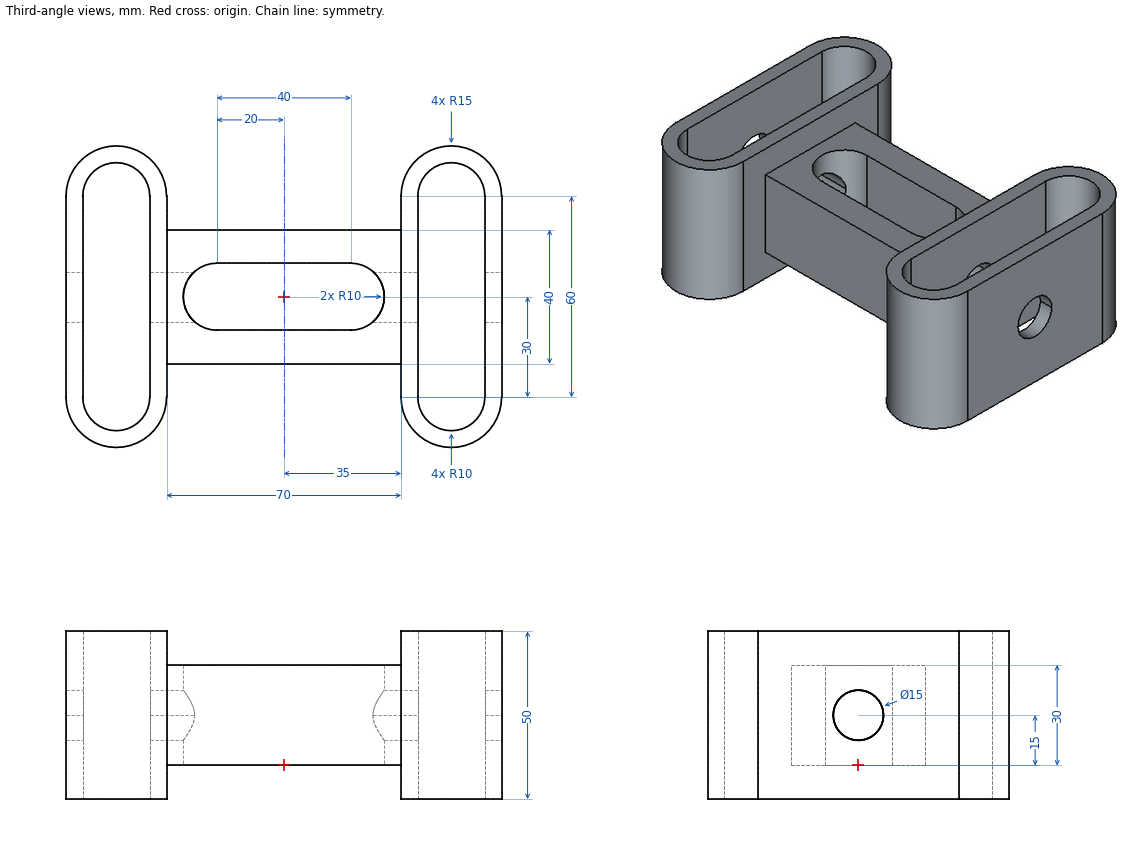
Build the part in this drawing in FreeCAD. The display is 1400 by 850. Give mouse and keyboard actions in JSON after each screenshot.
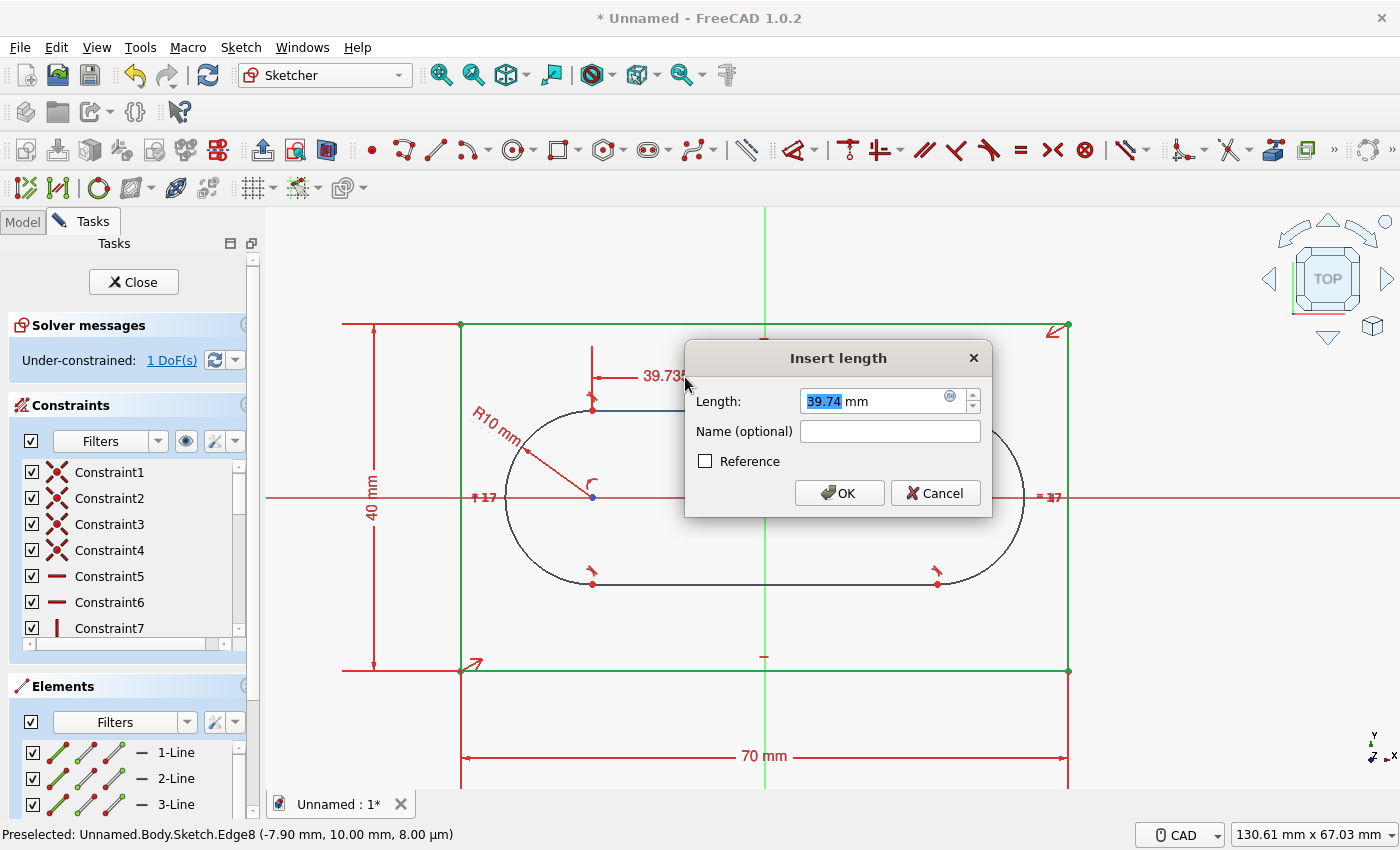
{"action": "type", "text": "40"}
{"action": "key", "text": "Return"}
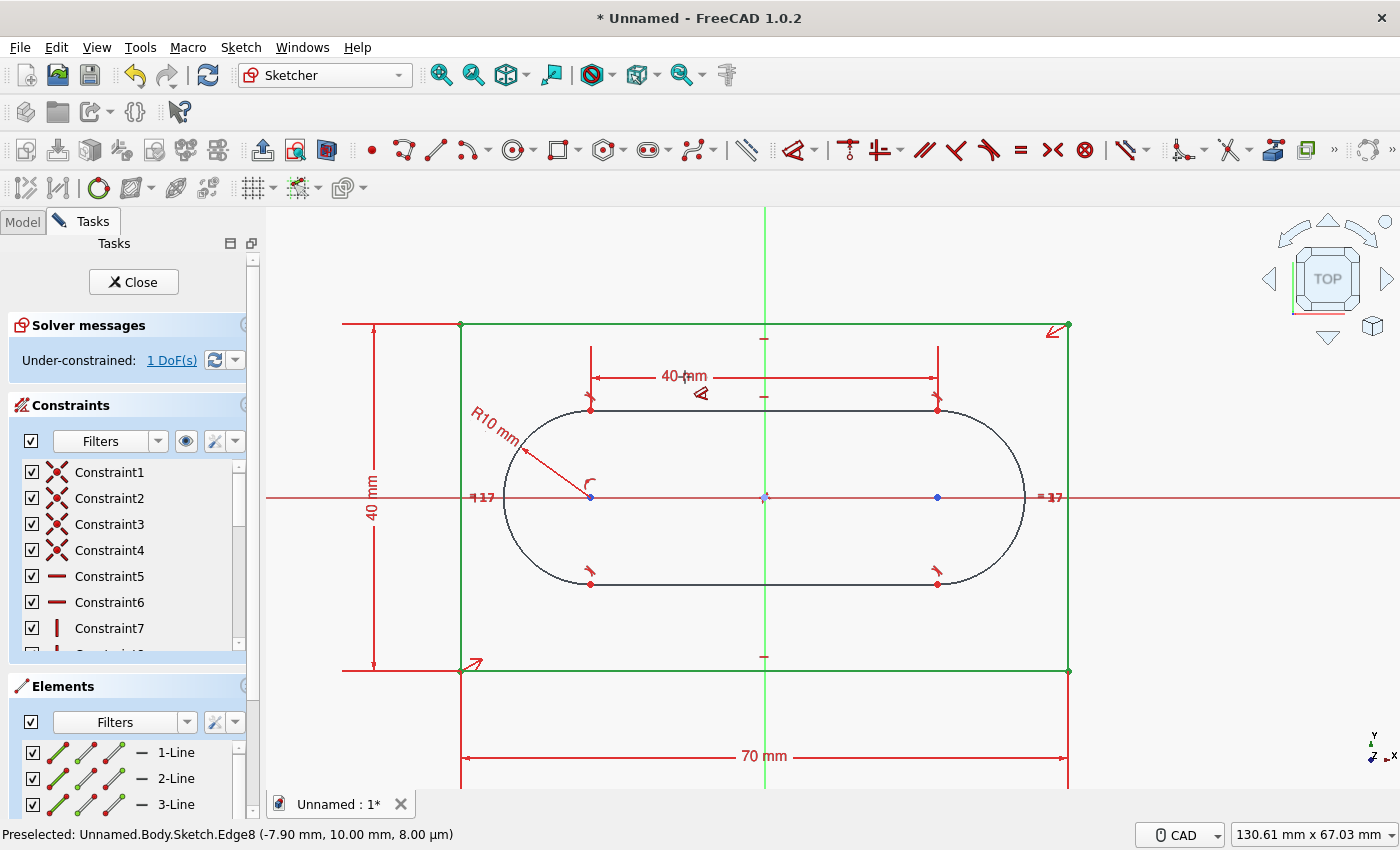
{"action": "left_click", "coordinate": [591, 411]}
{"action": "left_click", "coordinate": [678, 532]}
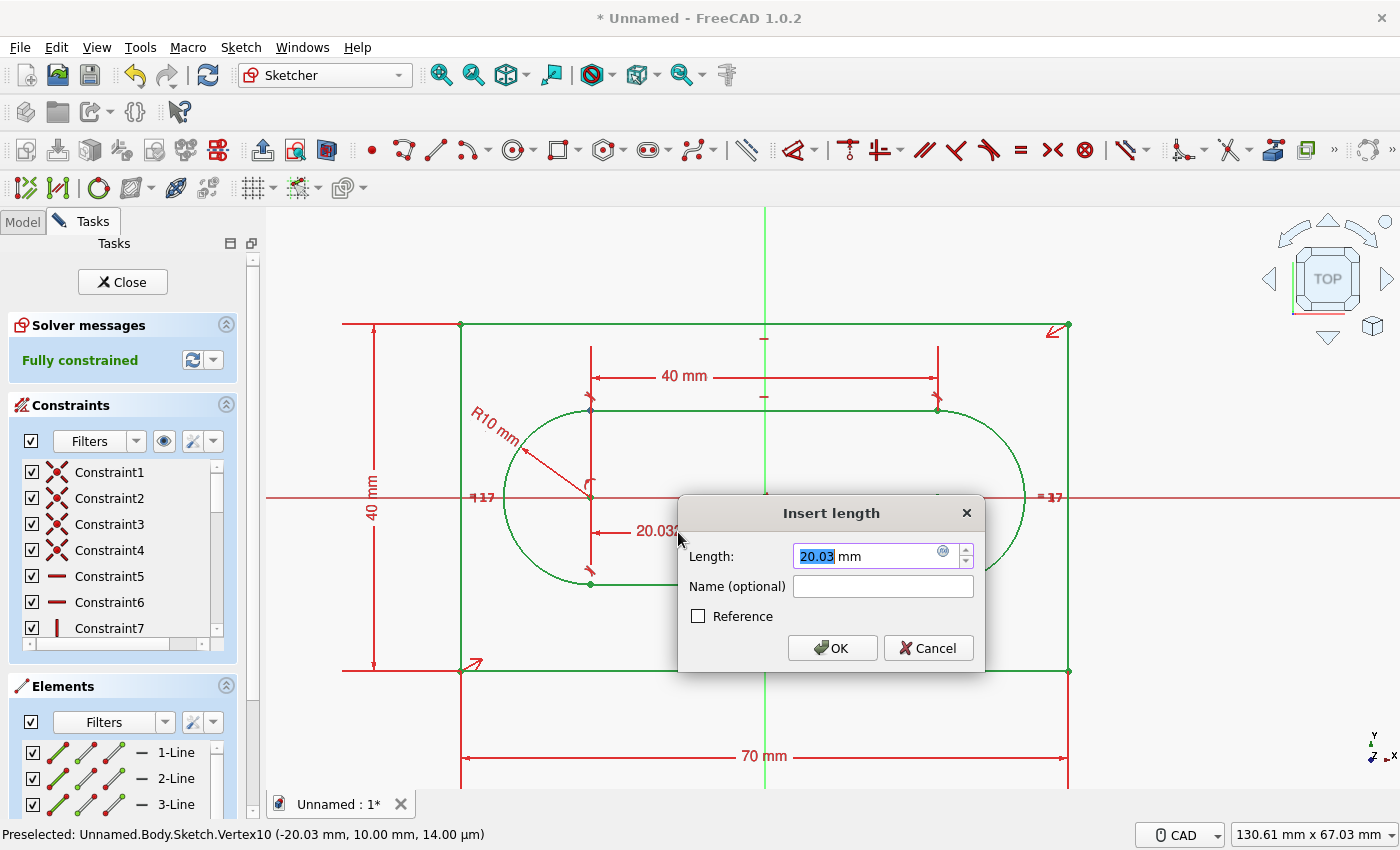
{"action": "type", "text": "20"}
{"action": "key", "text": "Return"}
{"action": "key", "text": "Escape"}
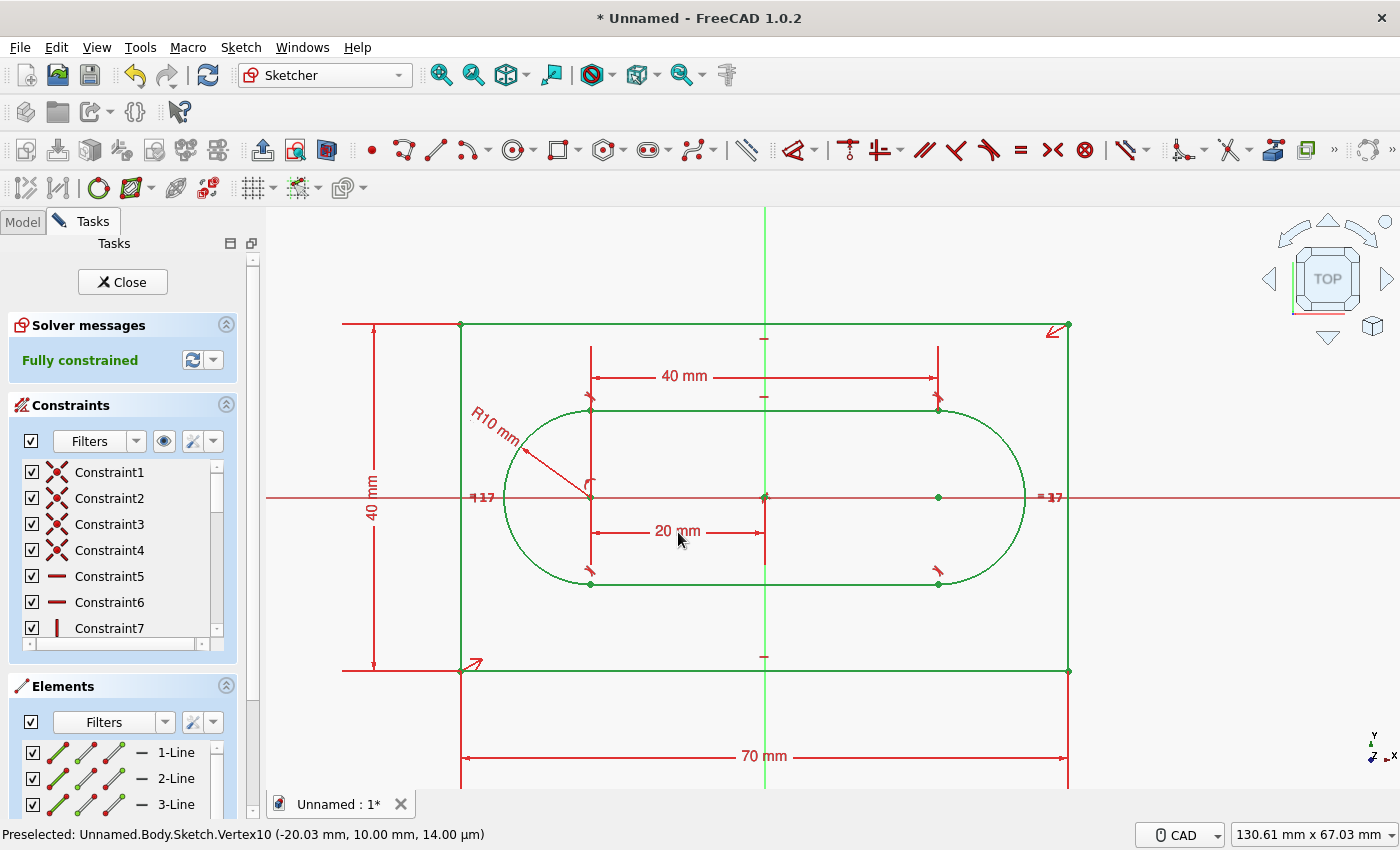
{"action": "left_click", "coordinate": [123, 282]}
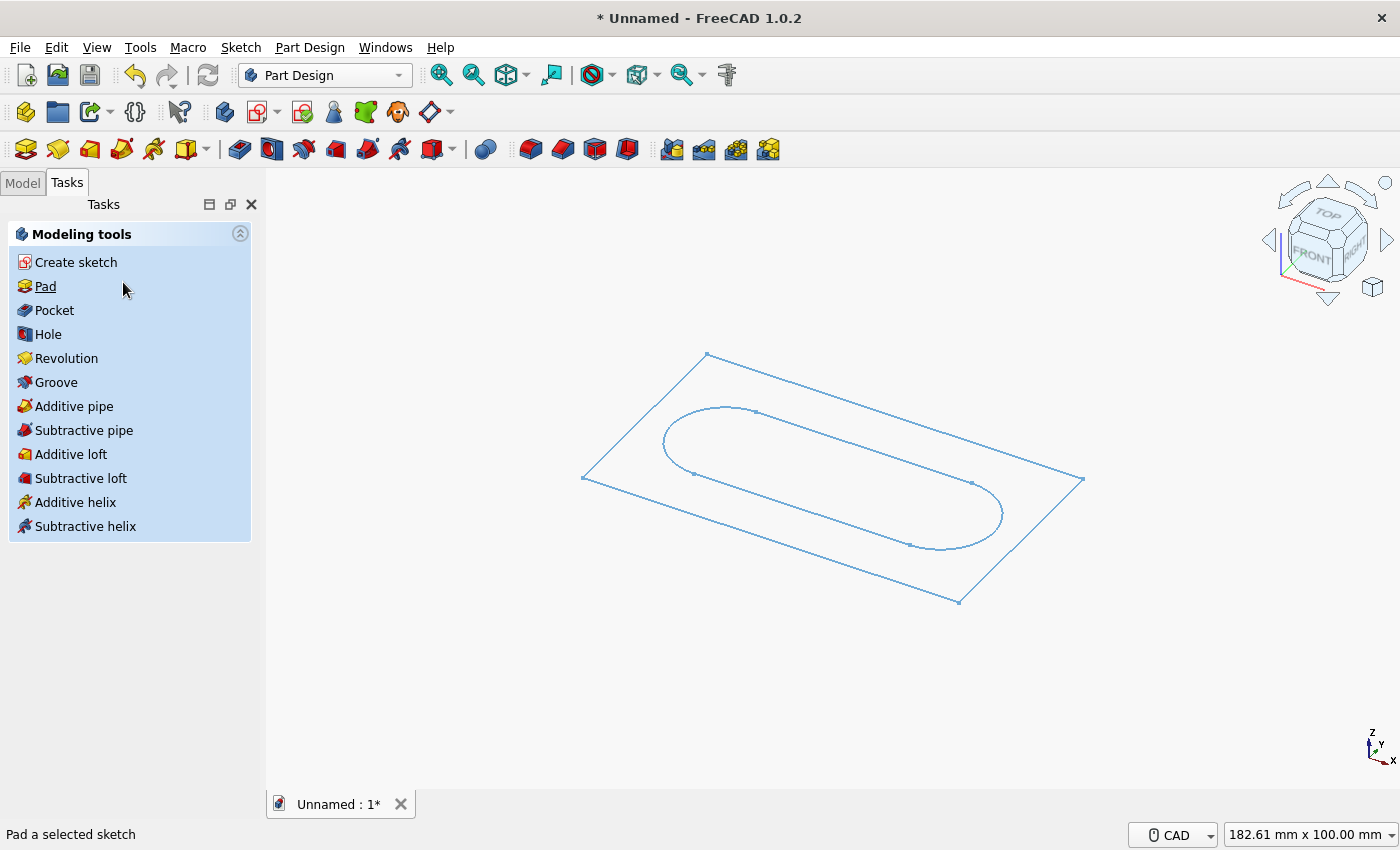
{"action": "left_click", "coordinate": [26, 150]}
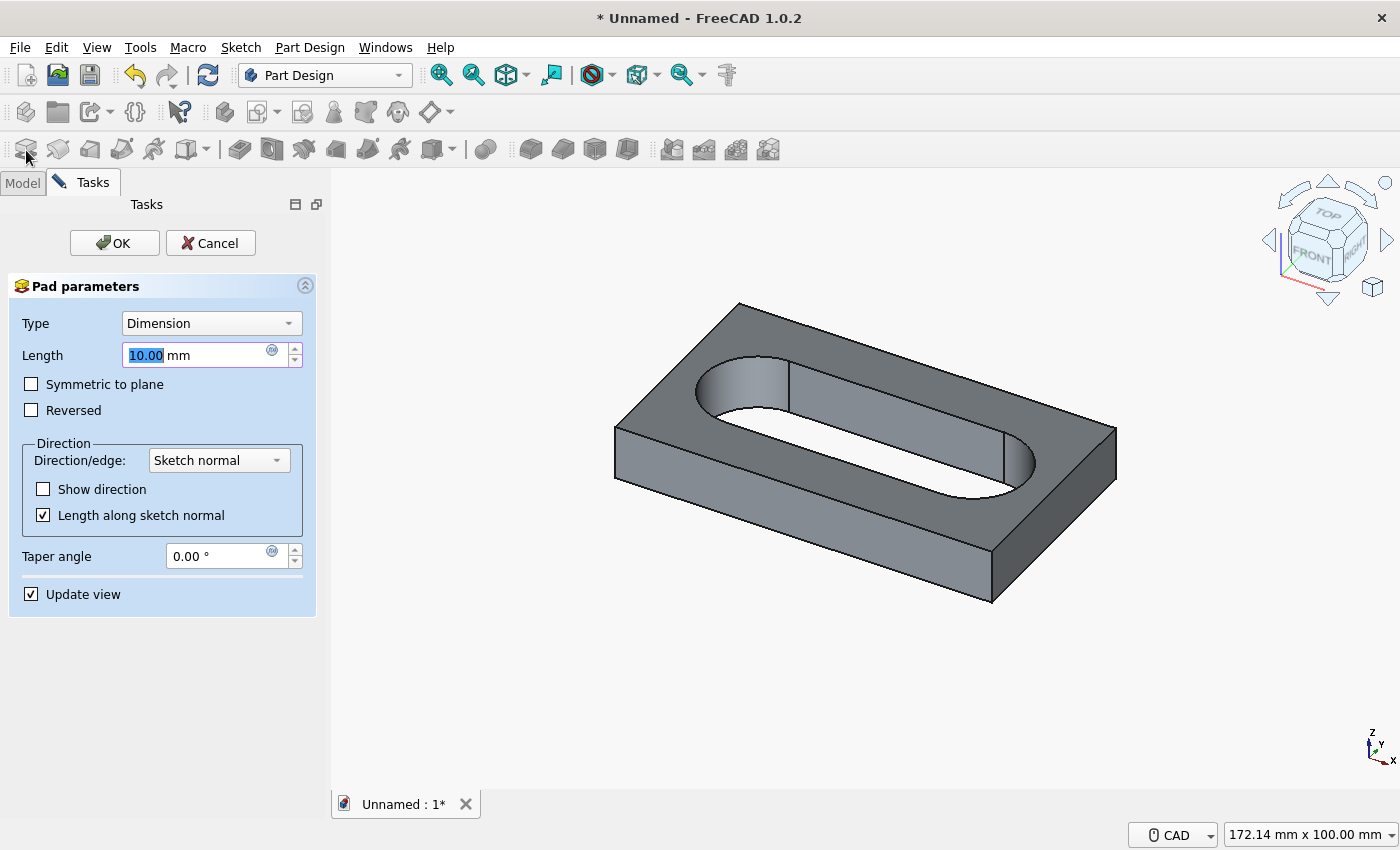
{"action": "type", "text": "30"}
{"action": "key", "text": "Tab"}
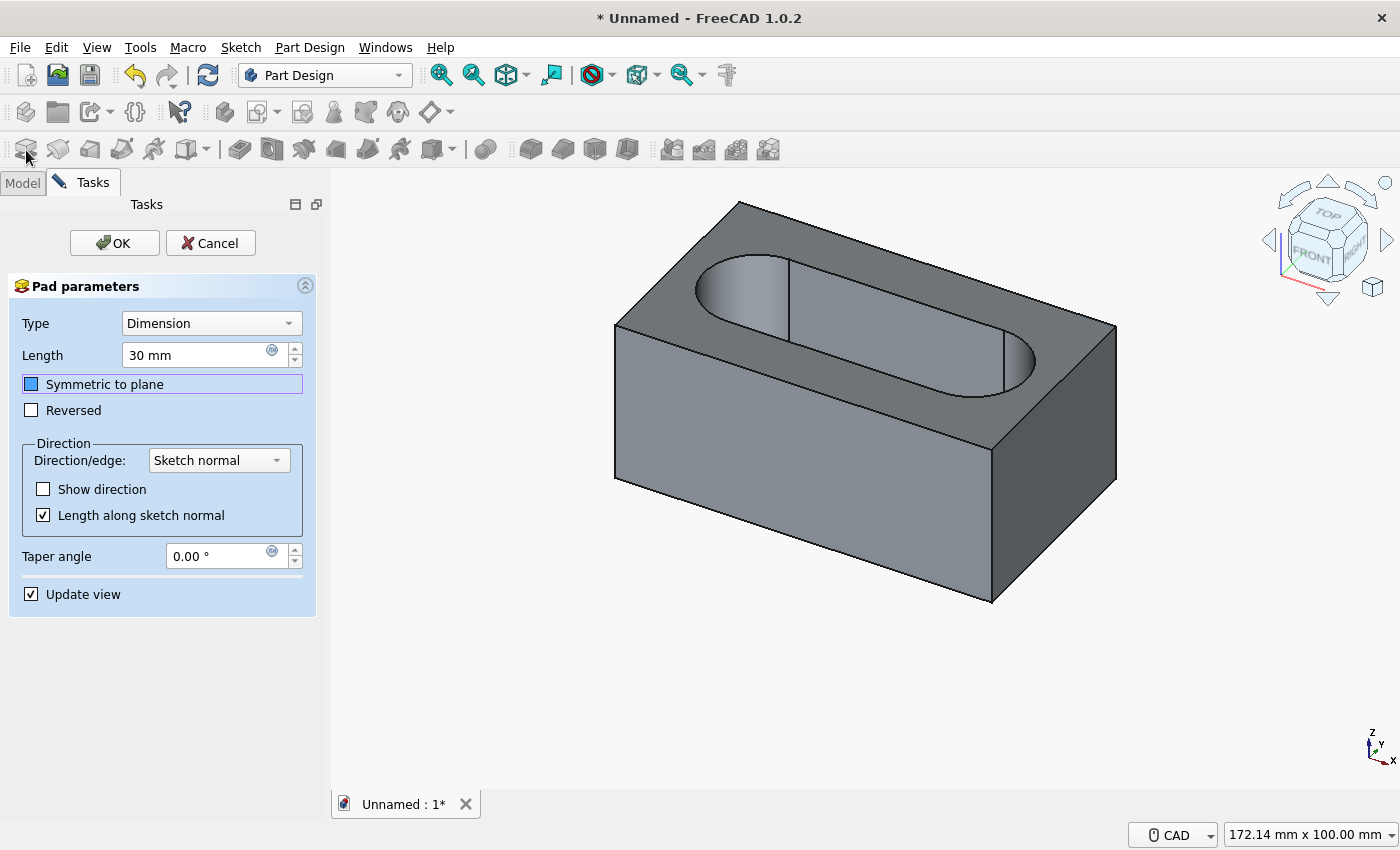
{"action": "left_click", "coordinate": [115, 243]}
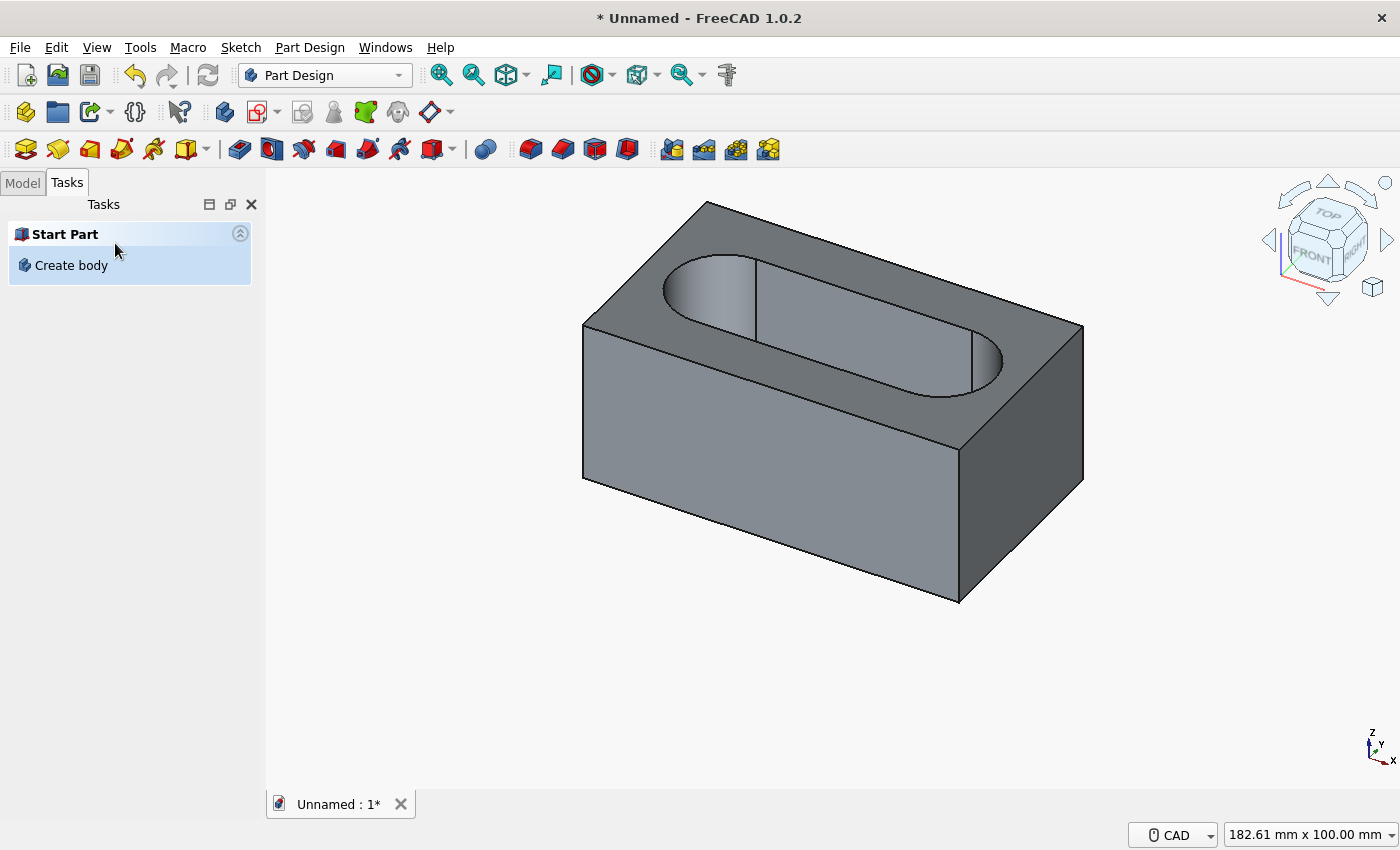
{"action": "left_click", "coordinate": [23, 182]}